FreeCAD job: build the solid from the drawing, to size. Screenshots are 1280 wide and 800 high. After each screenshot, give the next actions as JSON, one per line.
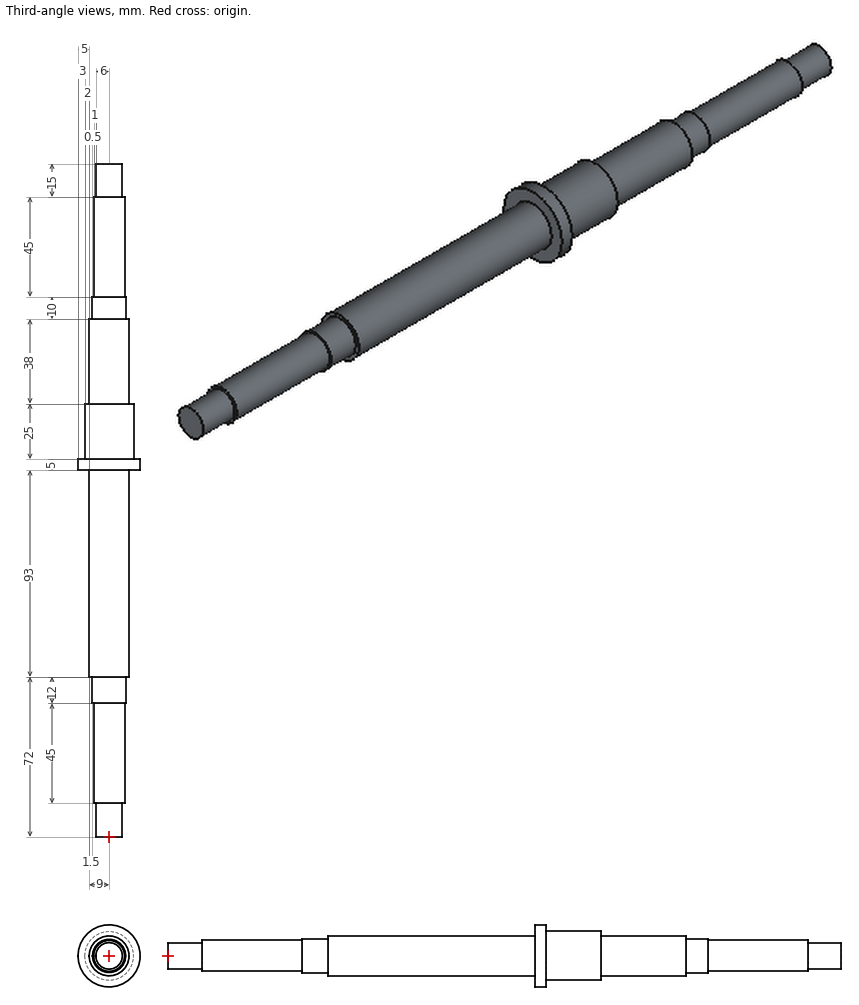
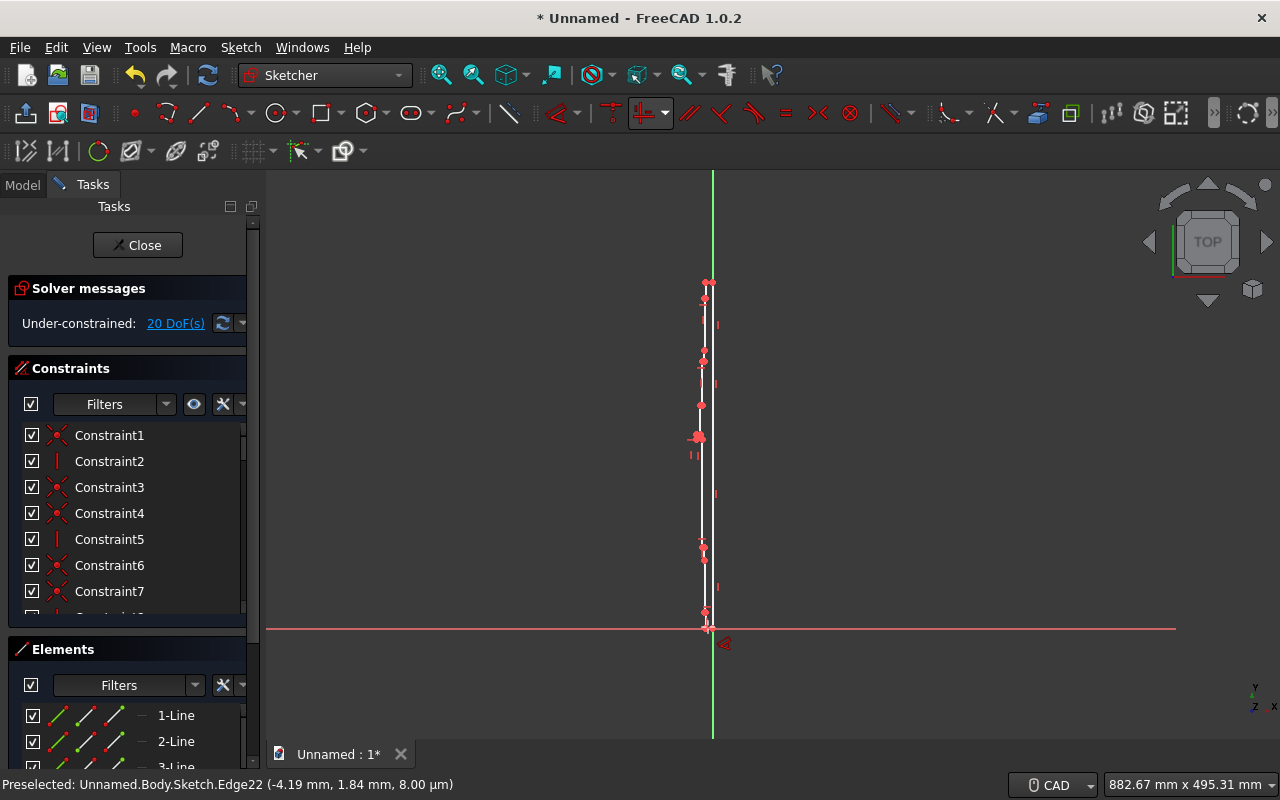
{"action": "scroll", "coordinate": [711, 282], "scroll_direction": "up", "scroll_amount": 10}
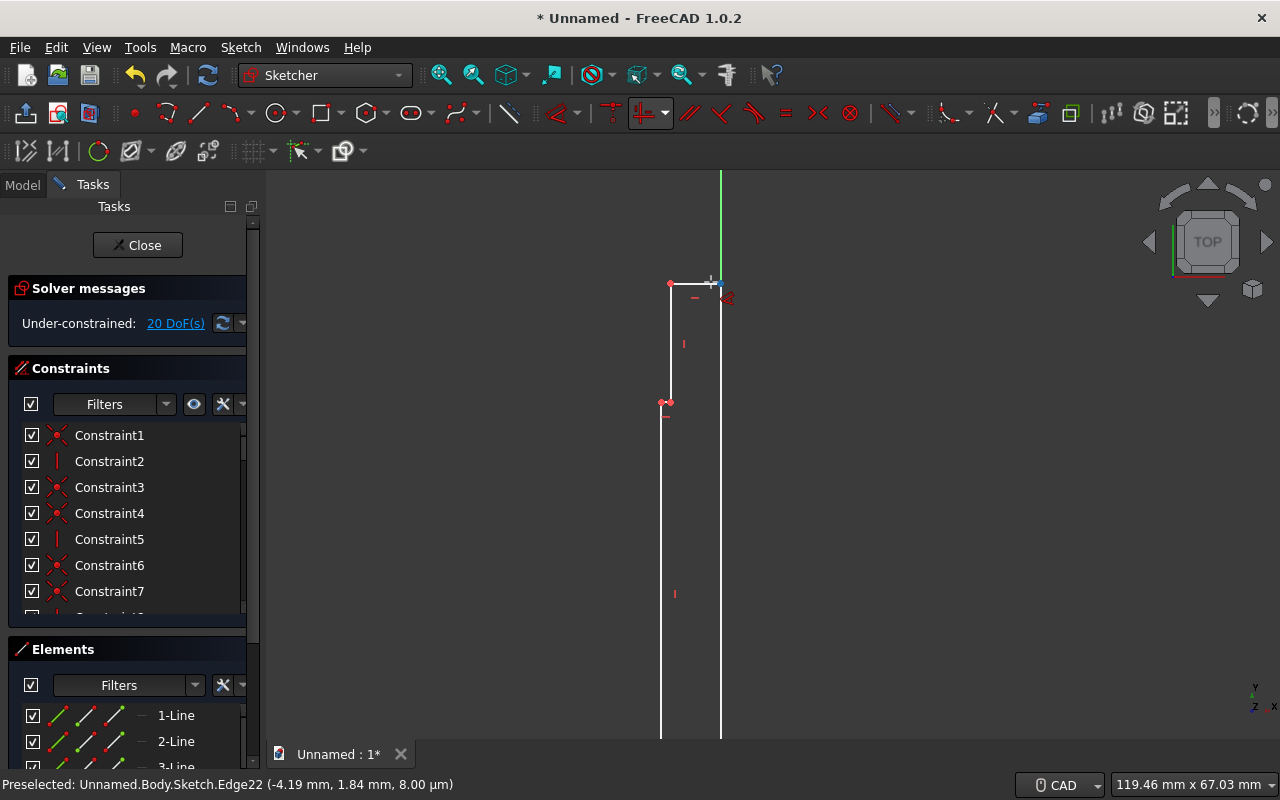
{"action": "left_click", "coordinate": [706, 284]}
{"action": "left_click", "coordinate": [696, 250]}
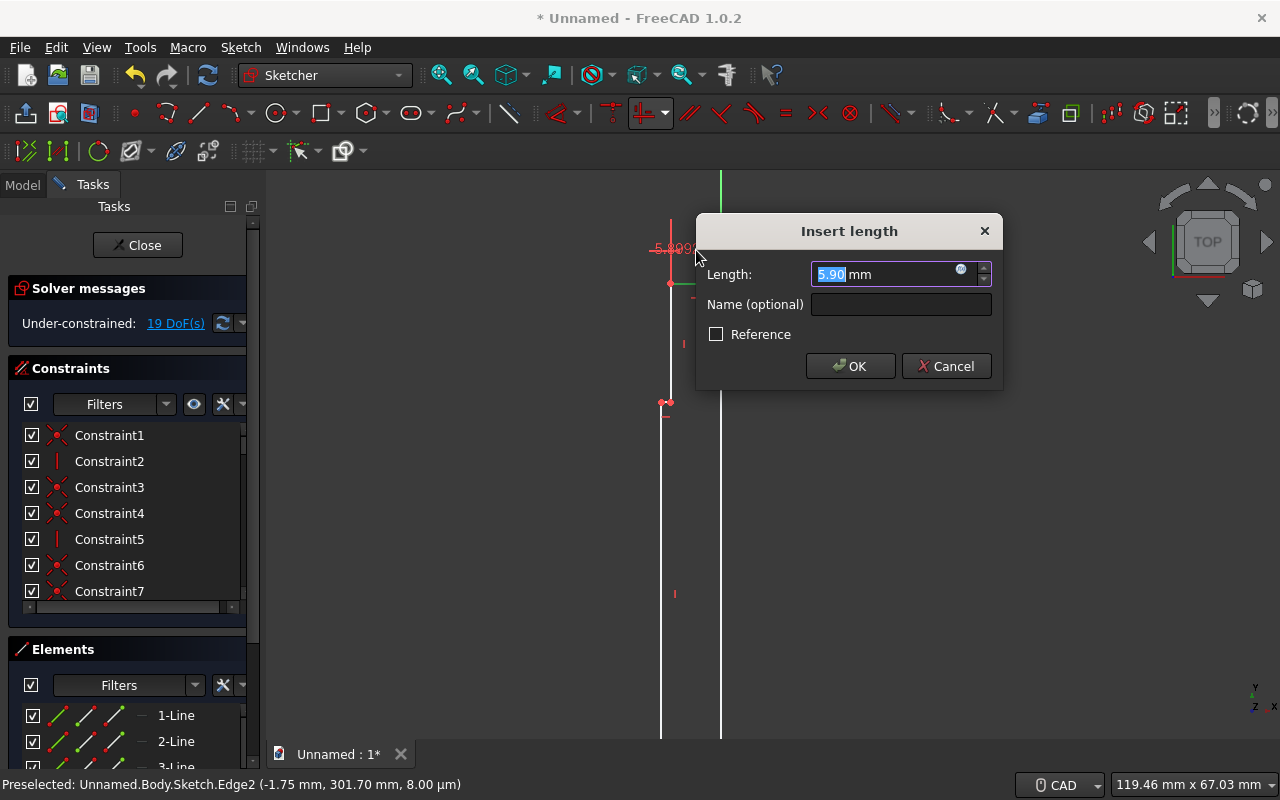
{"action": "type", "text": "6"}
{"action": "key", "text": "Return"}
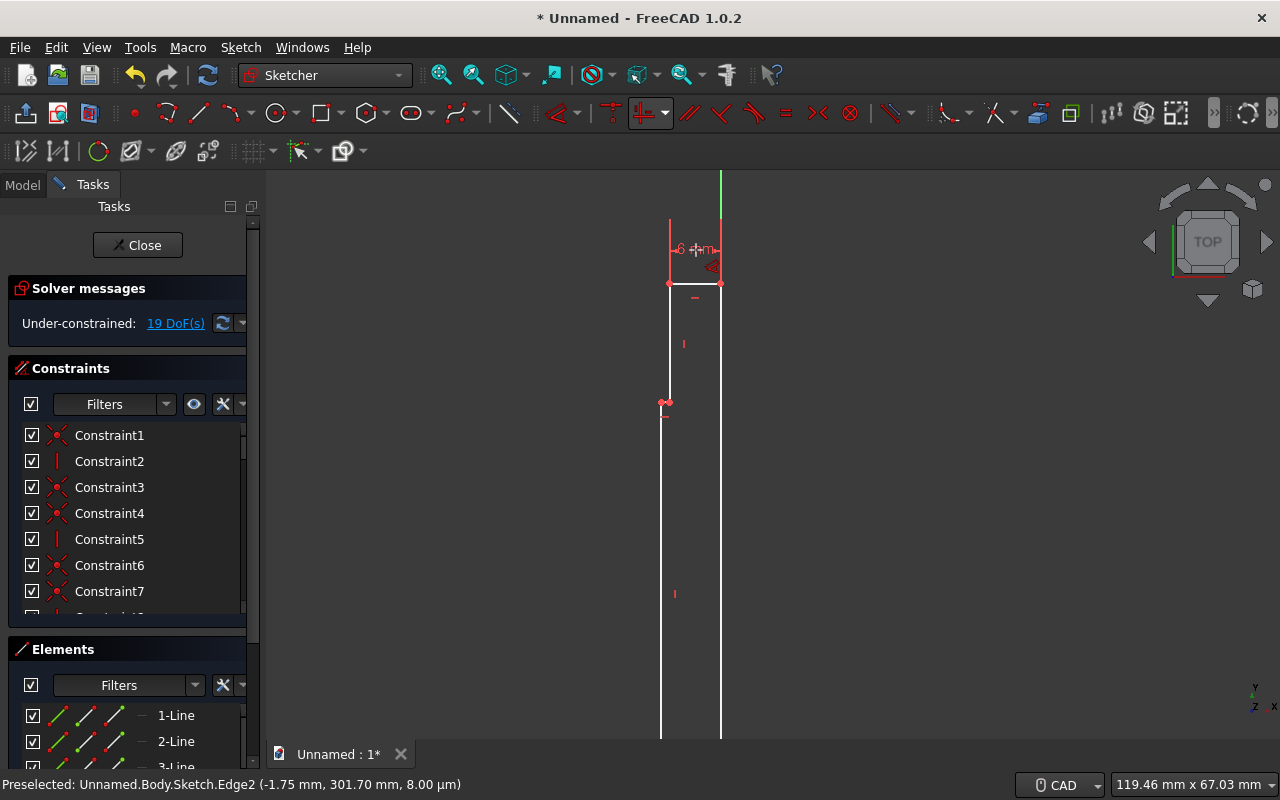
{"action": "scroll", "coordinate": [666, 402], "scroll_direction": "up", "scroll_amount": 8}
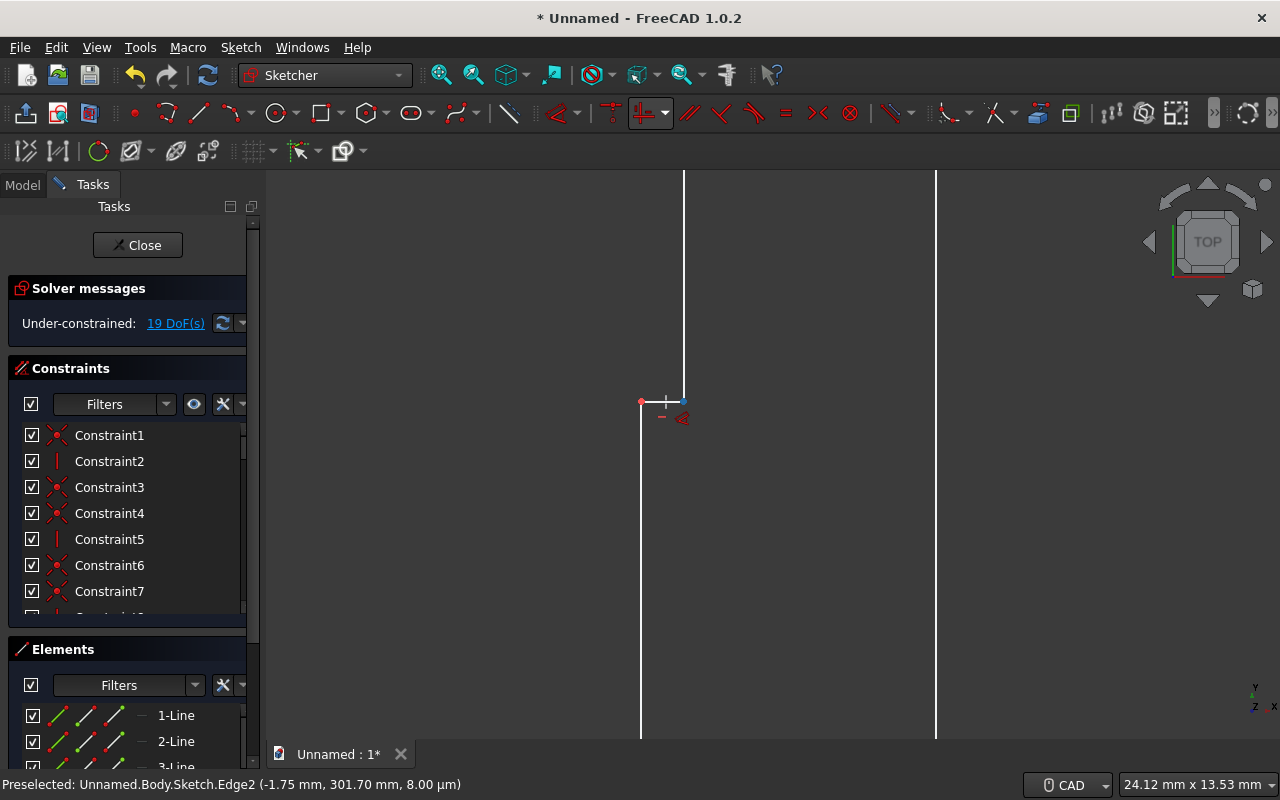
{"action": "left_click", "coordinate": [662, 402]}
{"action": "left_click", "coordinate": [662, 368]}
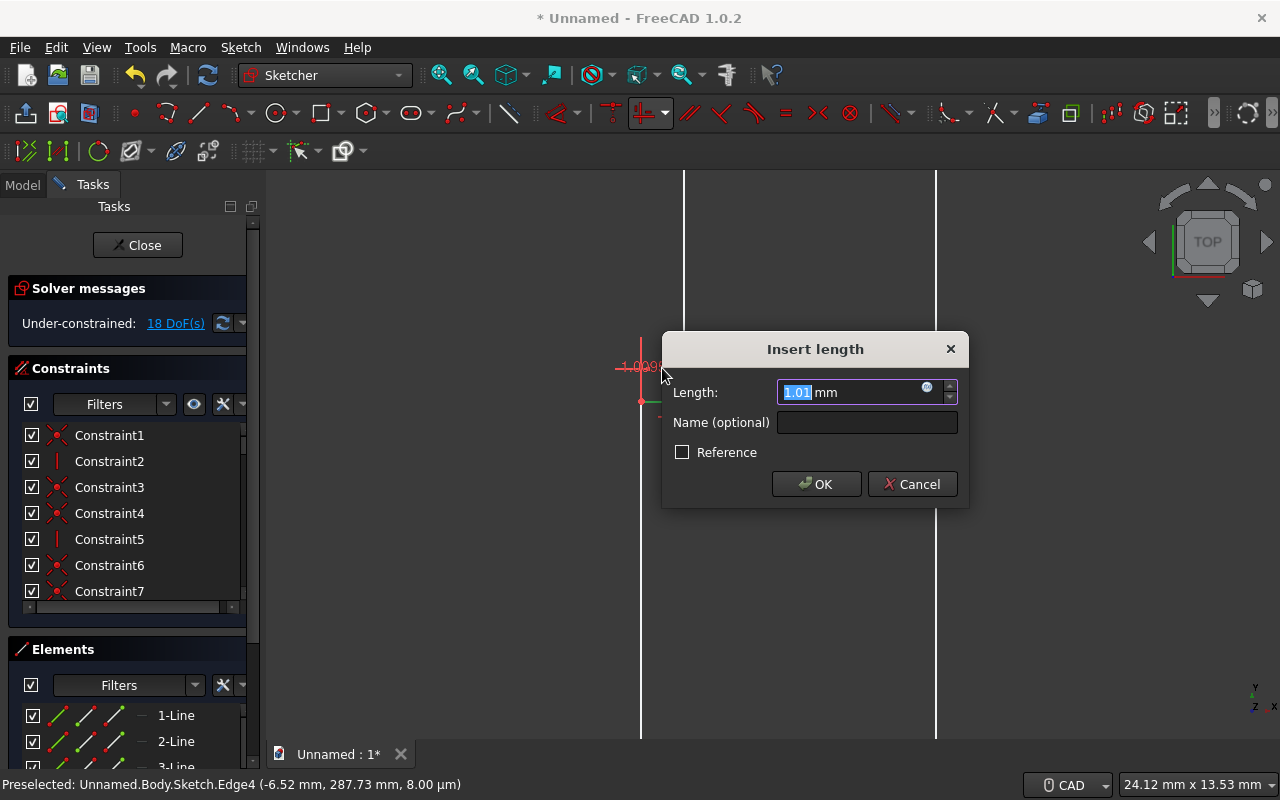
{"action": "type", "text": "1"}
{"action": "key", "text": "Return"}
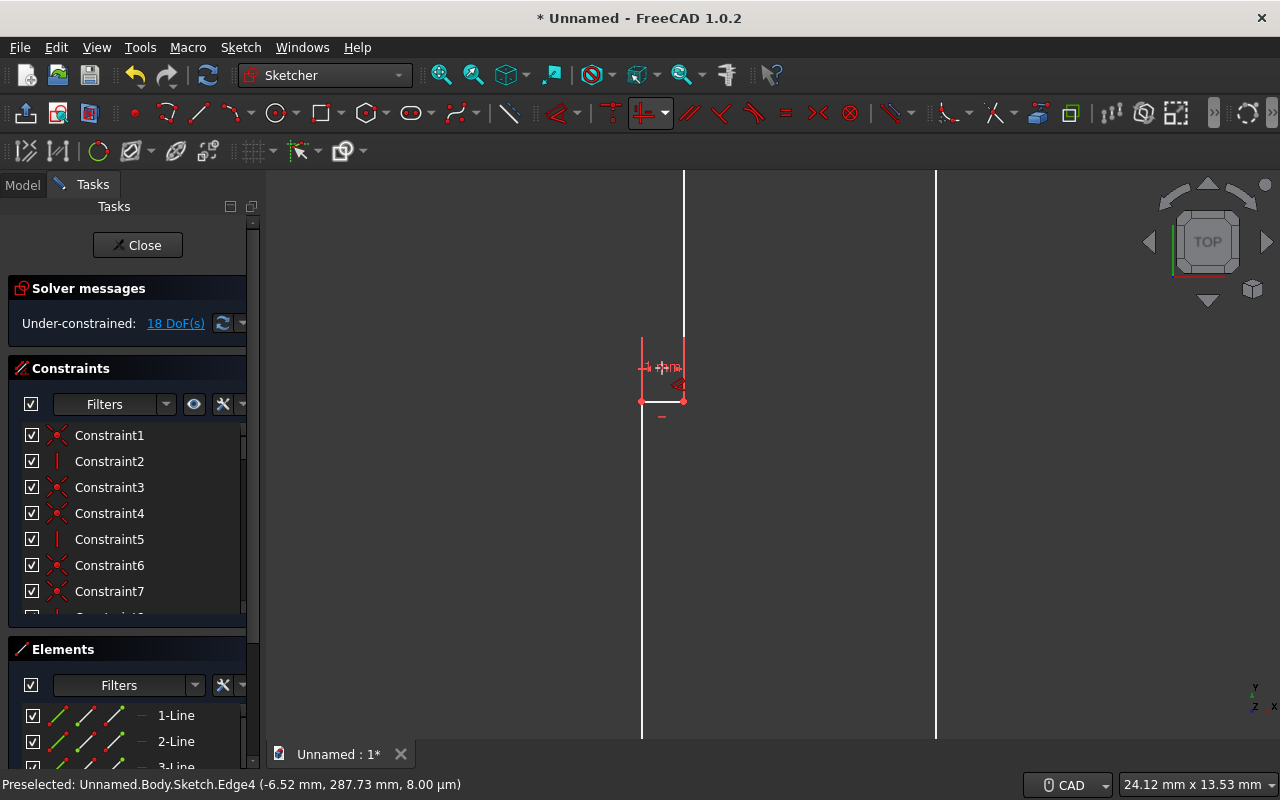
{"action": "scroll", "coordinate": [707, 259], "scroll_direction": "down", "scroll_amount": 17}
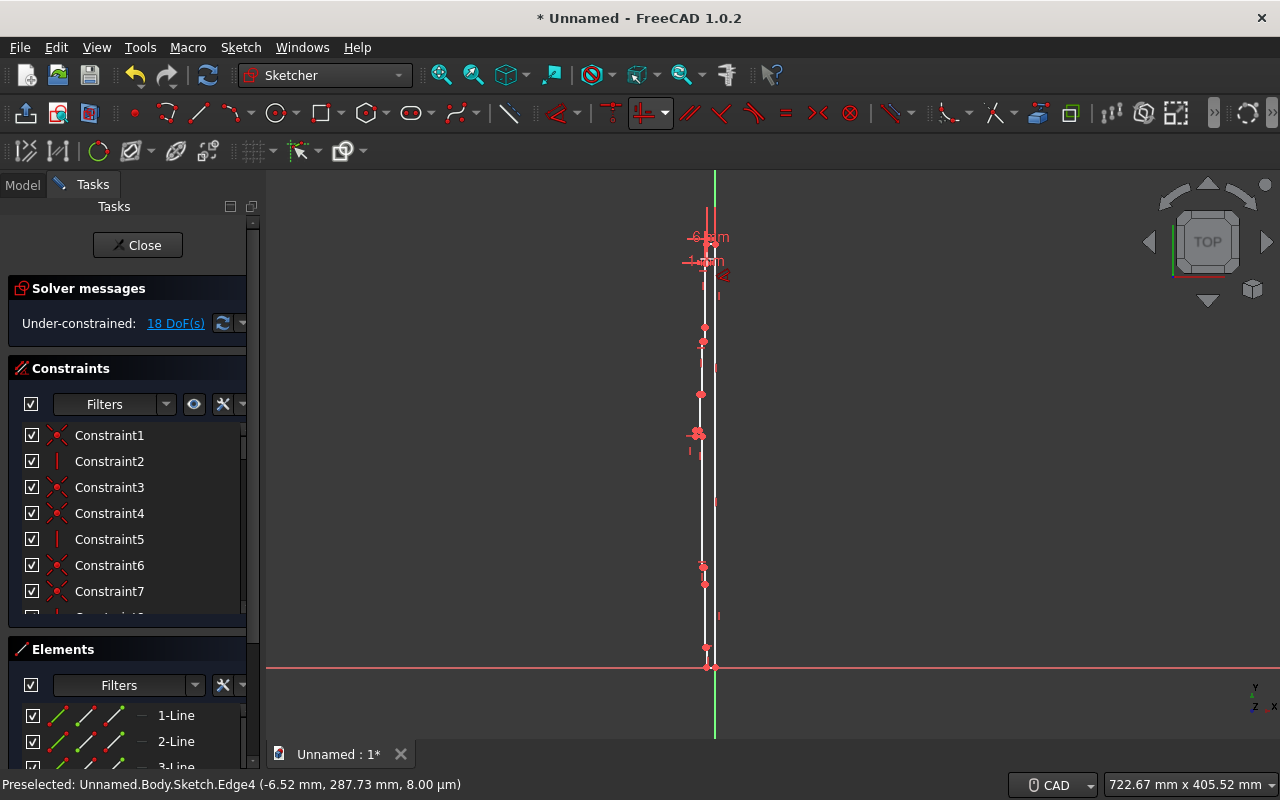
{"action": "scroll", "coordinate": [702, 395], "scroll_direction": "up", "scroll_amount": 14}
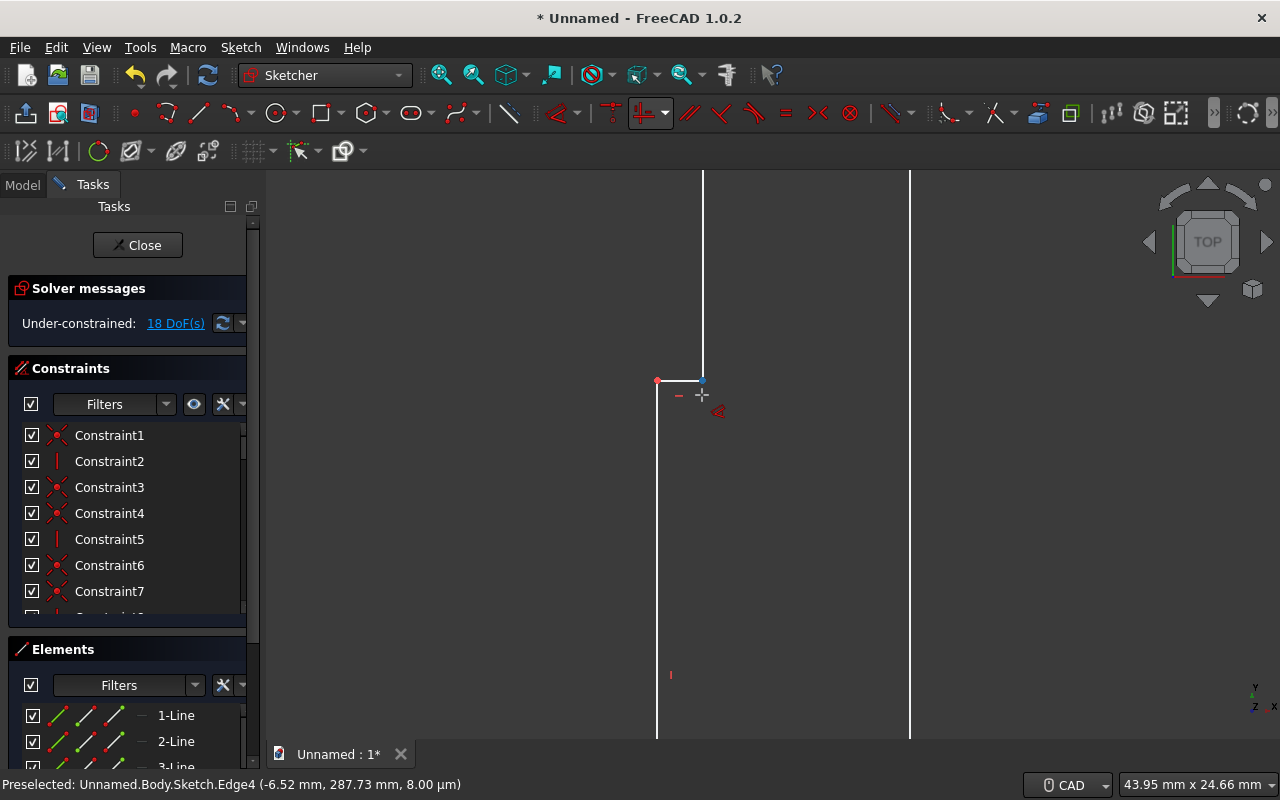
{"action": "left_click", "coordinate": [689, 381]}
{"action": "left_click", "coordinate": [680, 347]}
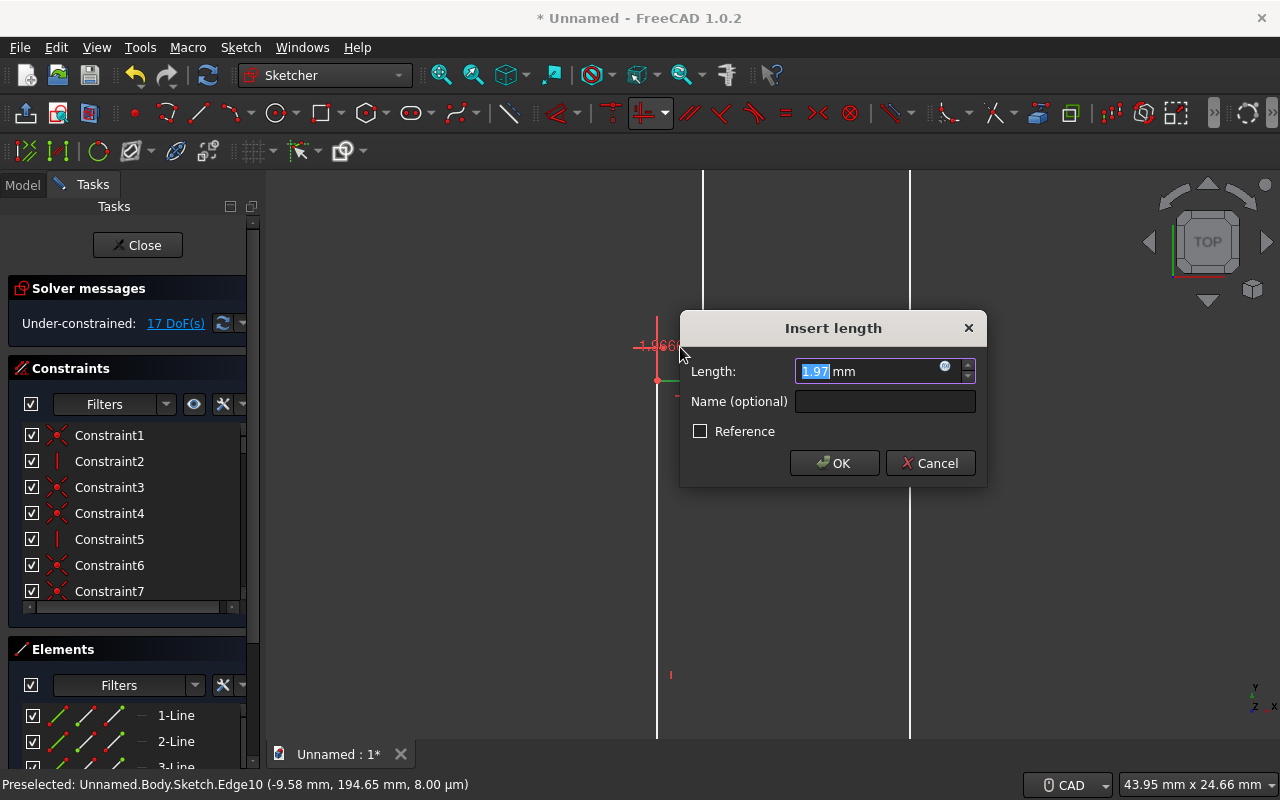
{"action": "type", "text": "2"}
{"action": "key", "text": "Return"}